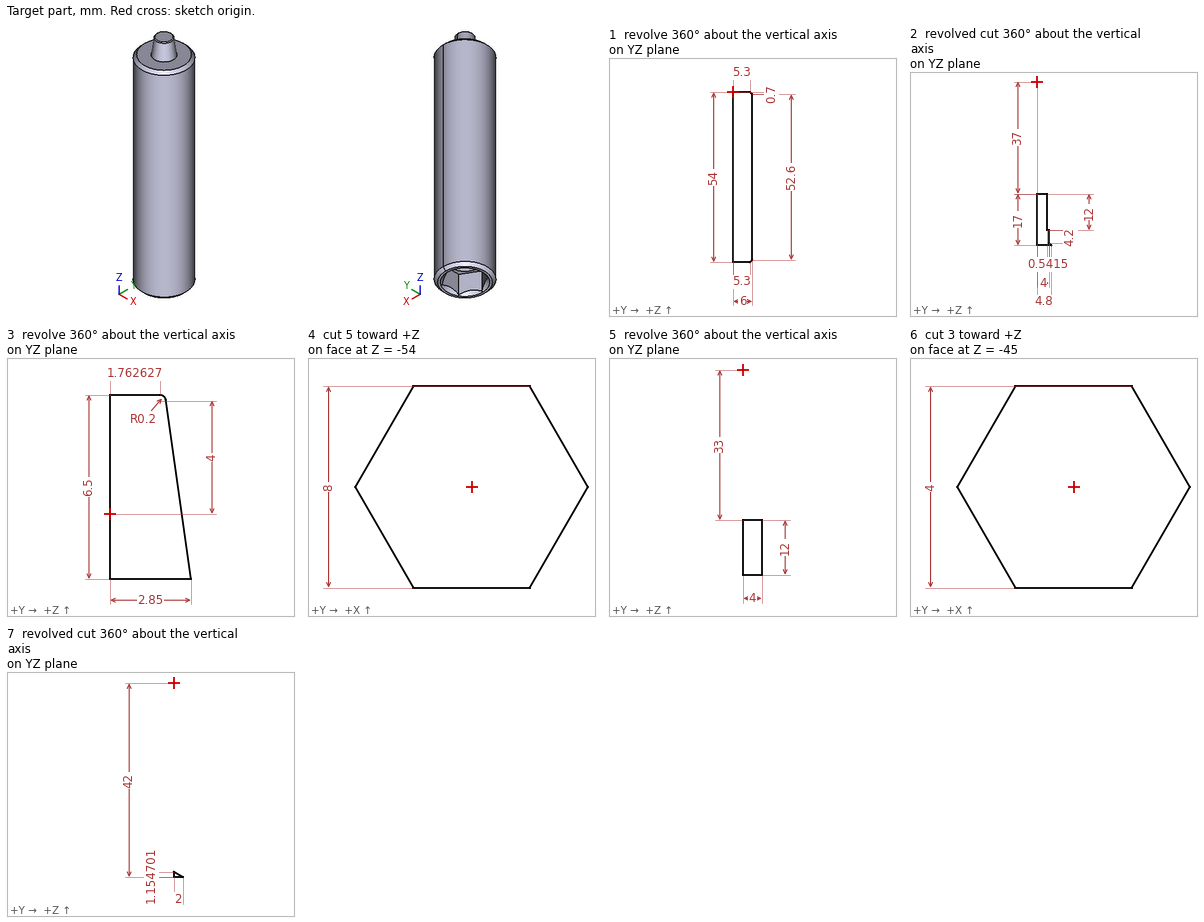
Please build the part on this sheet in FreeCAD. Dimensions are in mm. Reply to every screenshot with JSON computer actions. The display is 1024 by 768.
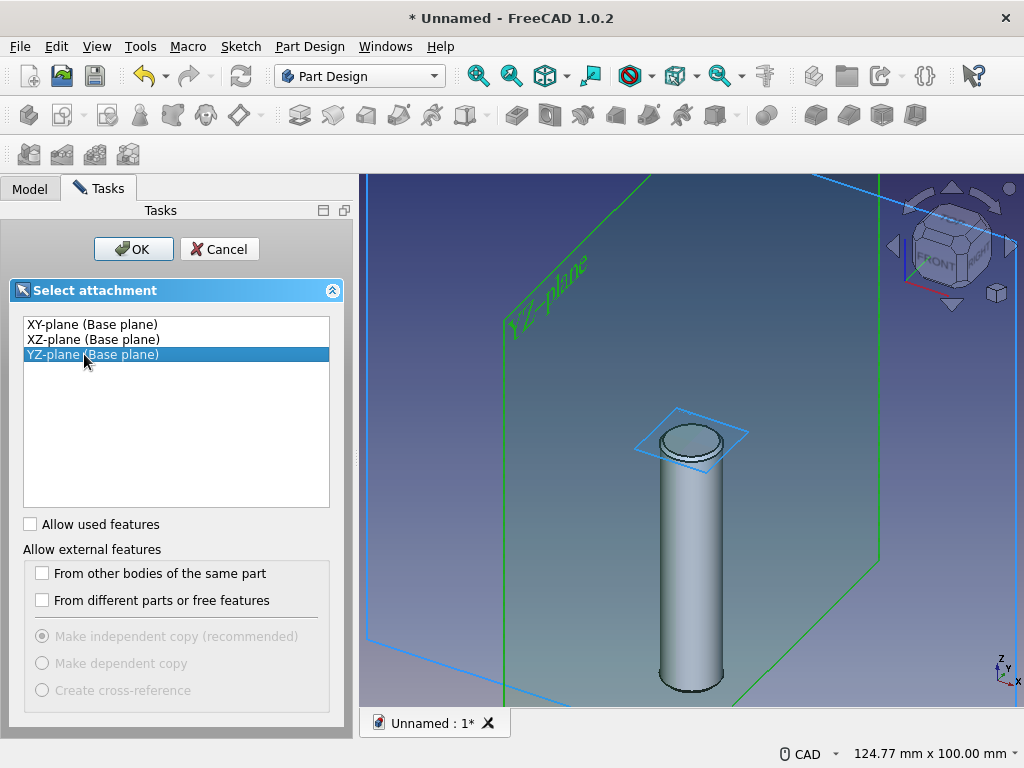
{"action": "left_click", "coordinate": [134, 249]}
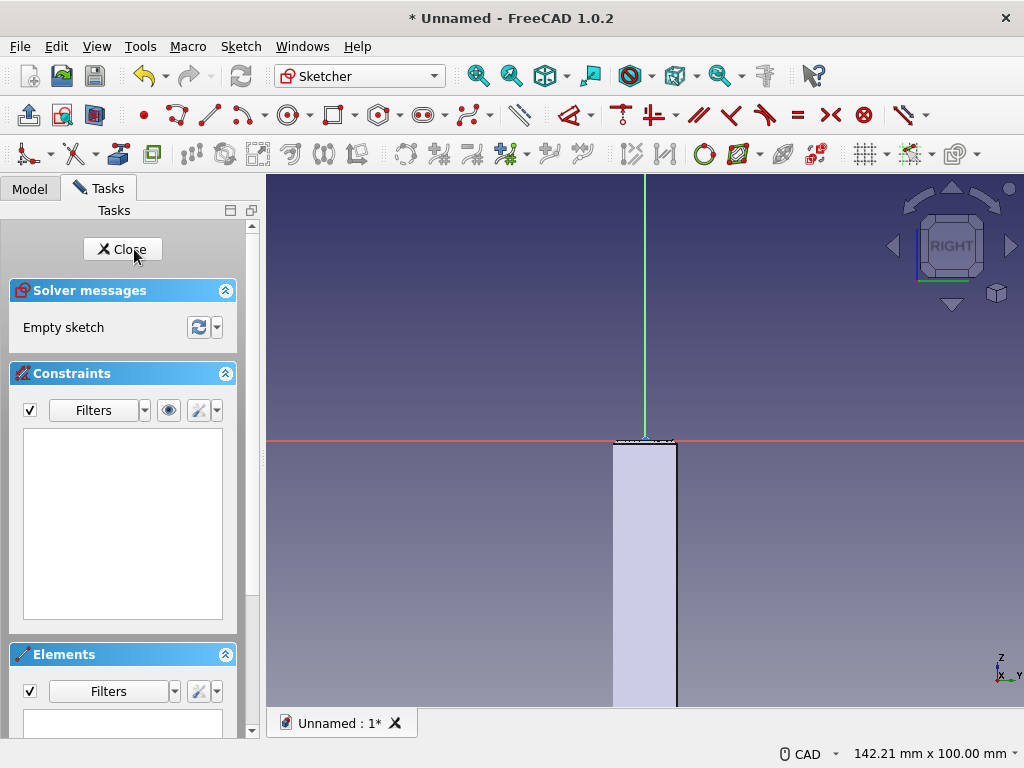
{"action": "left_click", "coordinate": [95, 116]}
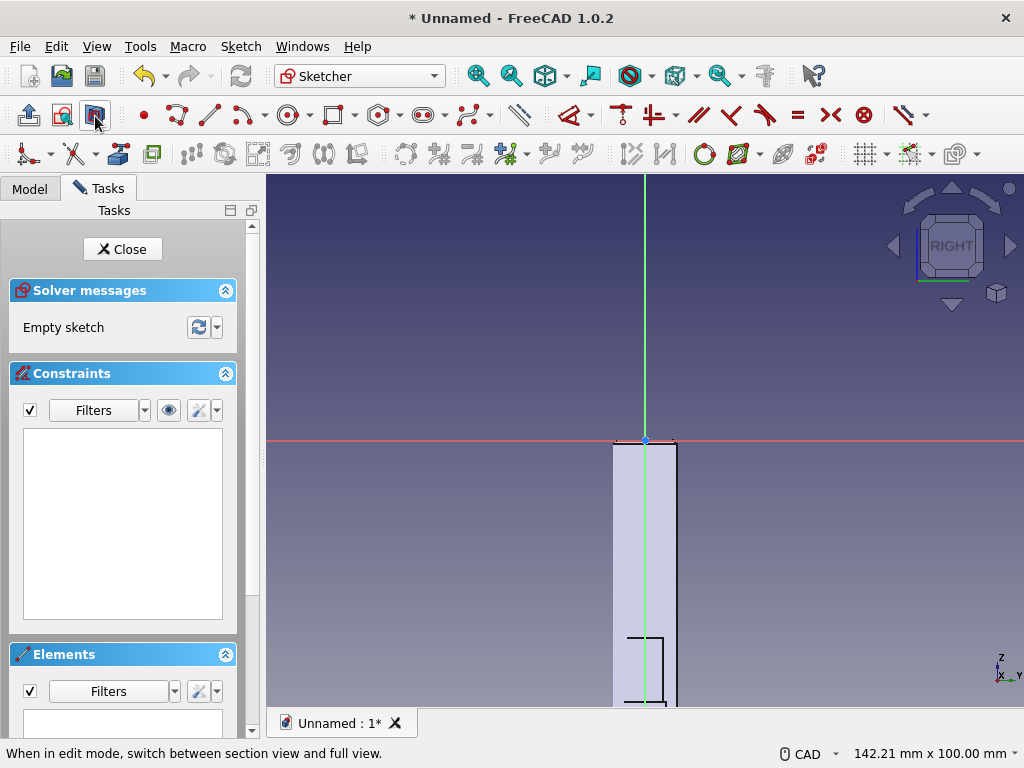
{"action": "scroll", "coordinate": [662, 435], "scroll_direction": "up", "scroll_amount": 11}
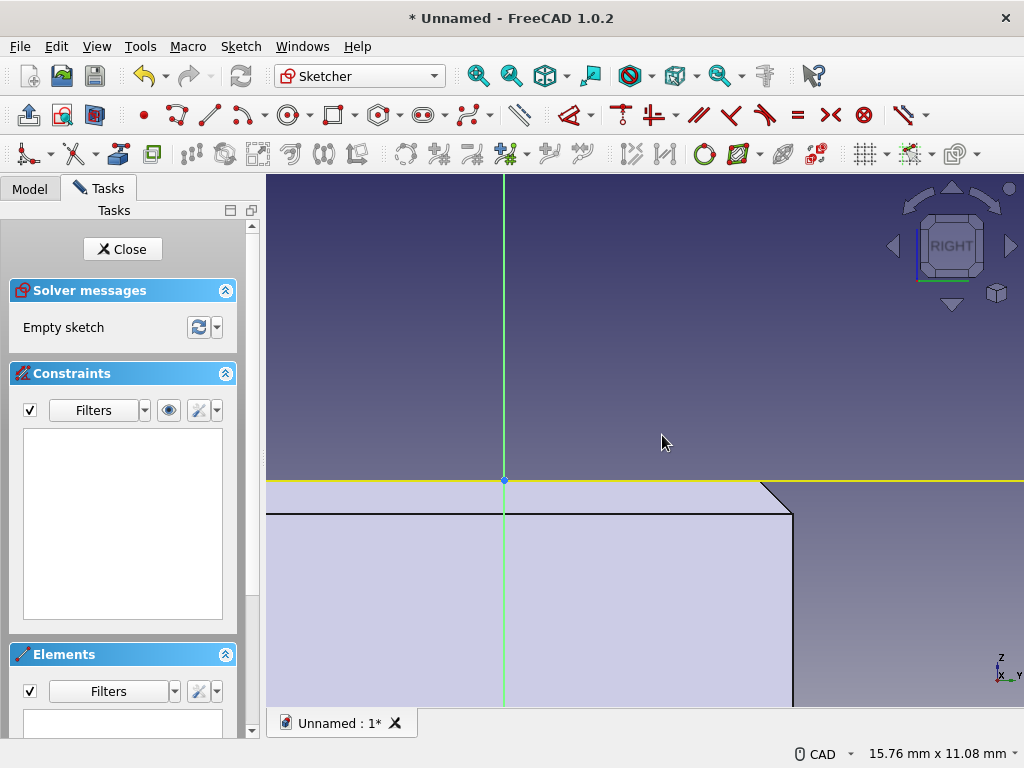
{"action": "left_click", "coordinate": [177, 116]}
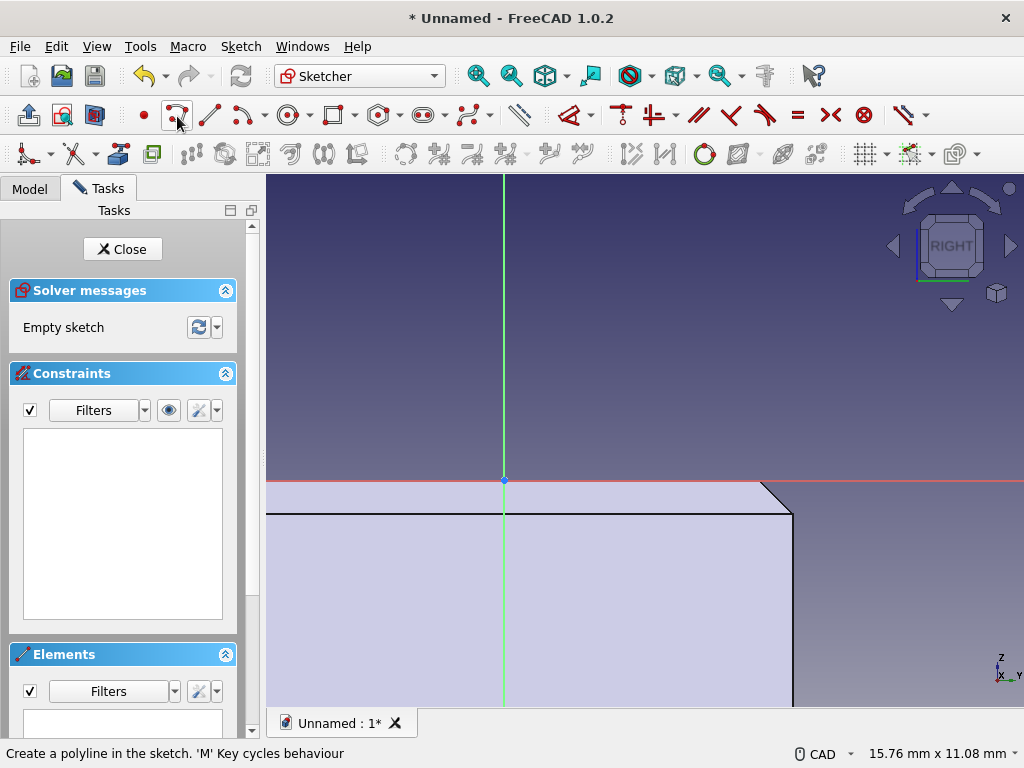
{"action": "left_click", "coordinate": [589, 279]}
{"action": "left_click", "coordinate": [504, 279]}
{"action": "left_click", "coordinate": [513, 591]}
{"action": "left_click", "coordinate": [641, 591]}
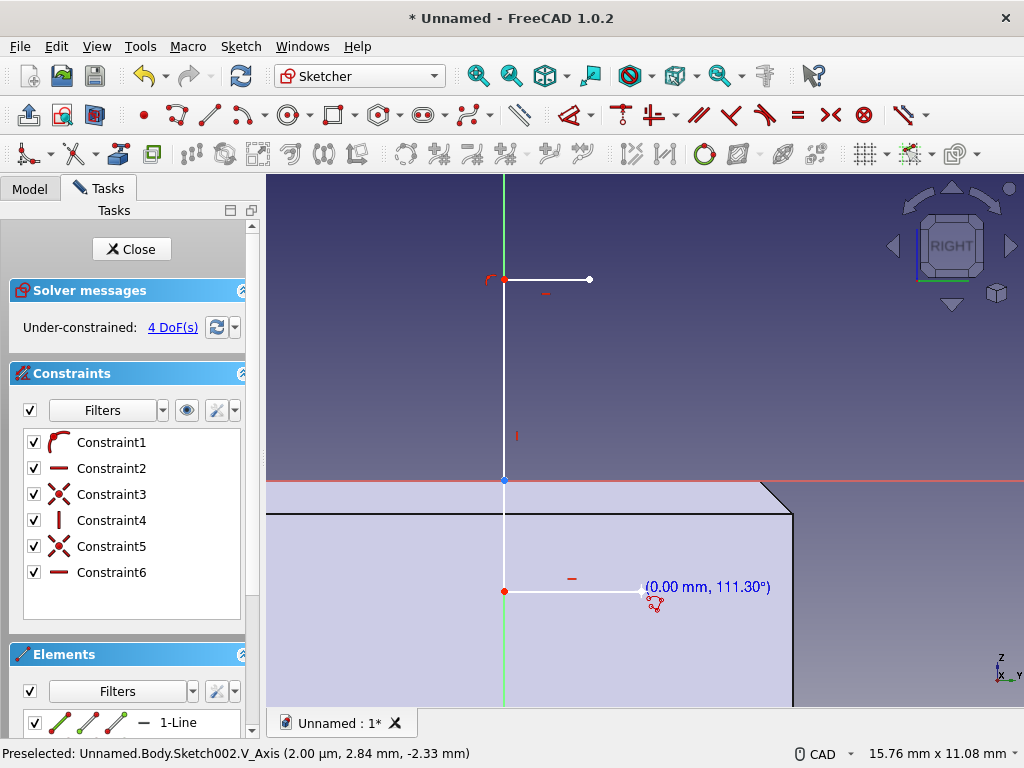
{"action": "scroll", "coordinate": [599, 287], "scroll_direction": "up", "scroll_amount": 2}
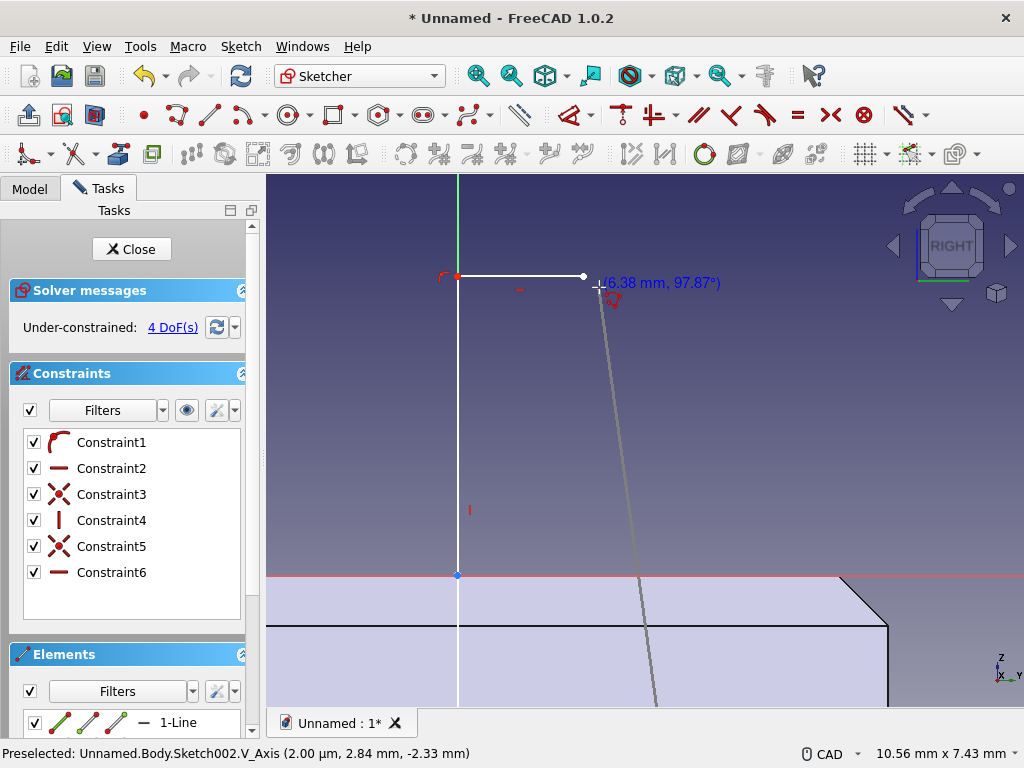
{"action": "left_click", "coordinate": [598, 287]}
{"action": "right_click", "coordinate": [598, 287]}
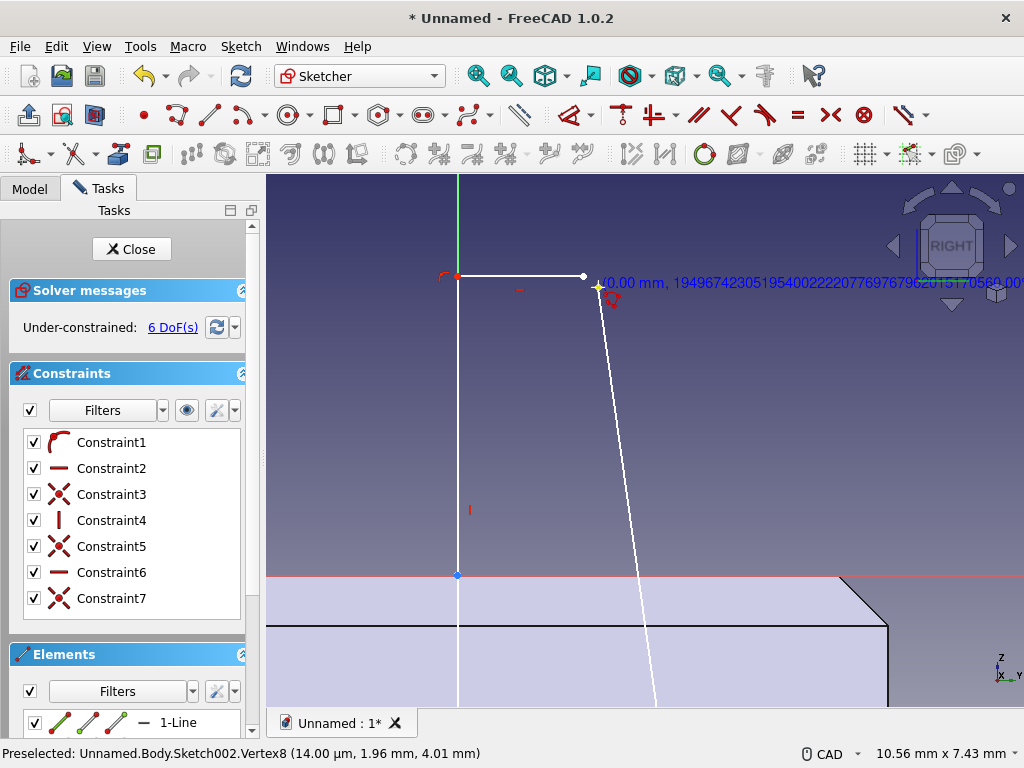
{"action": "left_click", "coordinate": [264, 116]}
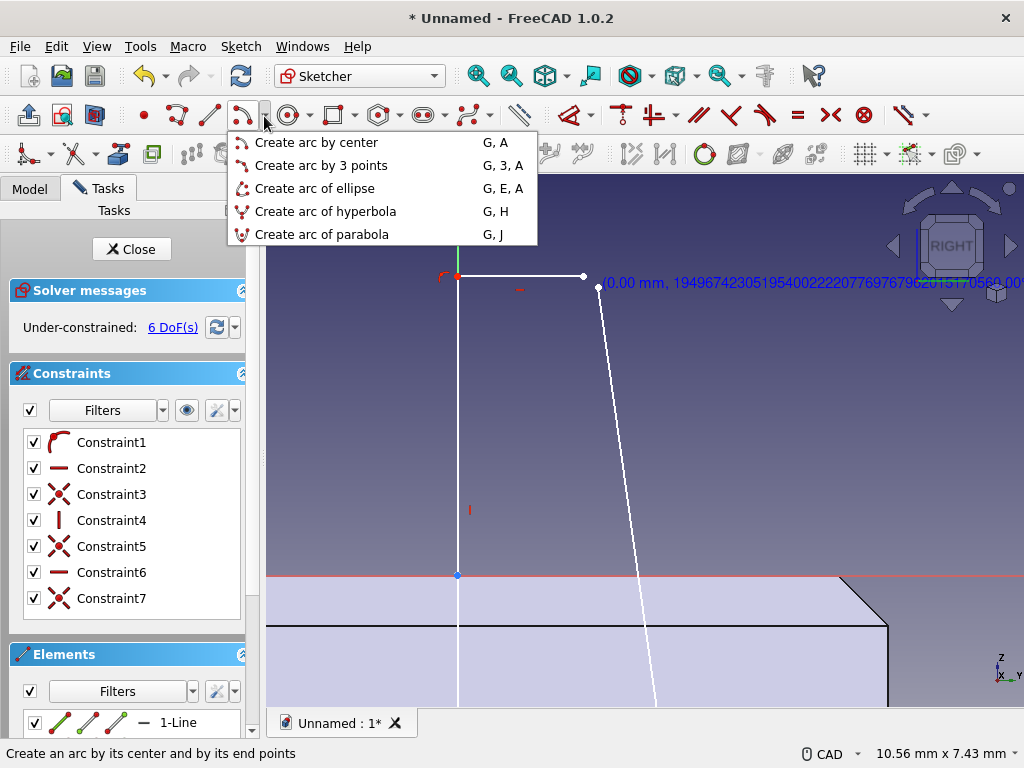
{"action": "left_click", "coordinate": [382, 166]}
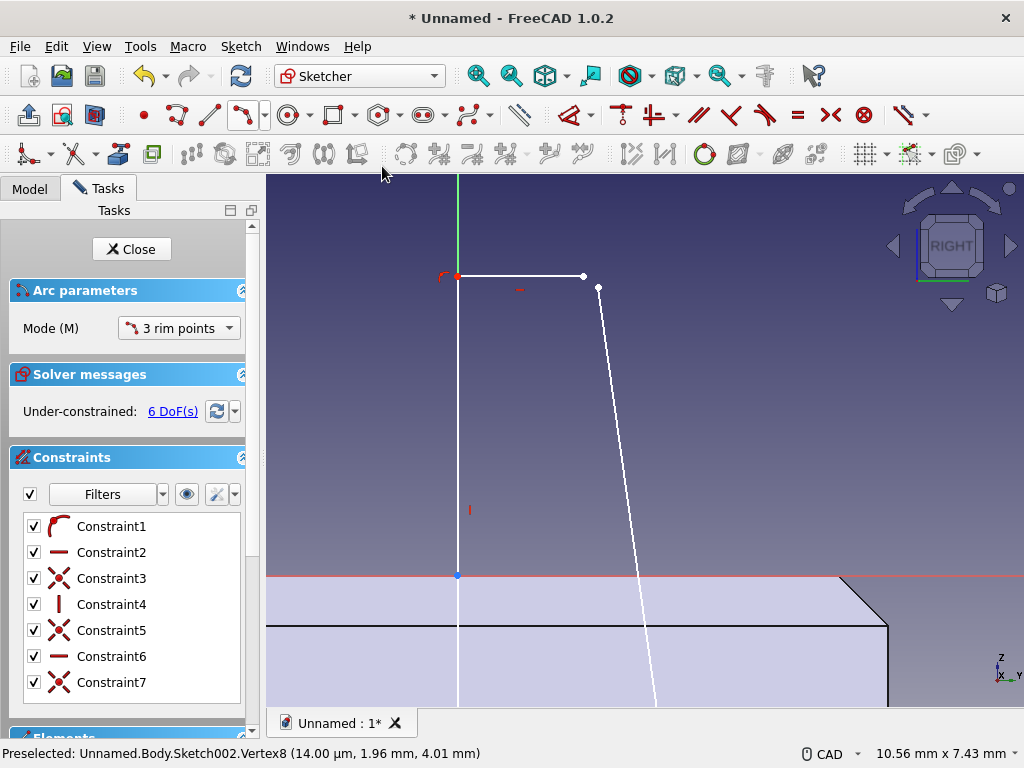
{"action": "left_click", "coordinate": [598, 288]}
{"action": "left_click", "coordinate": [584, 276]}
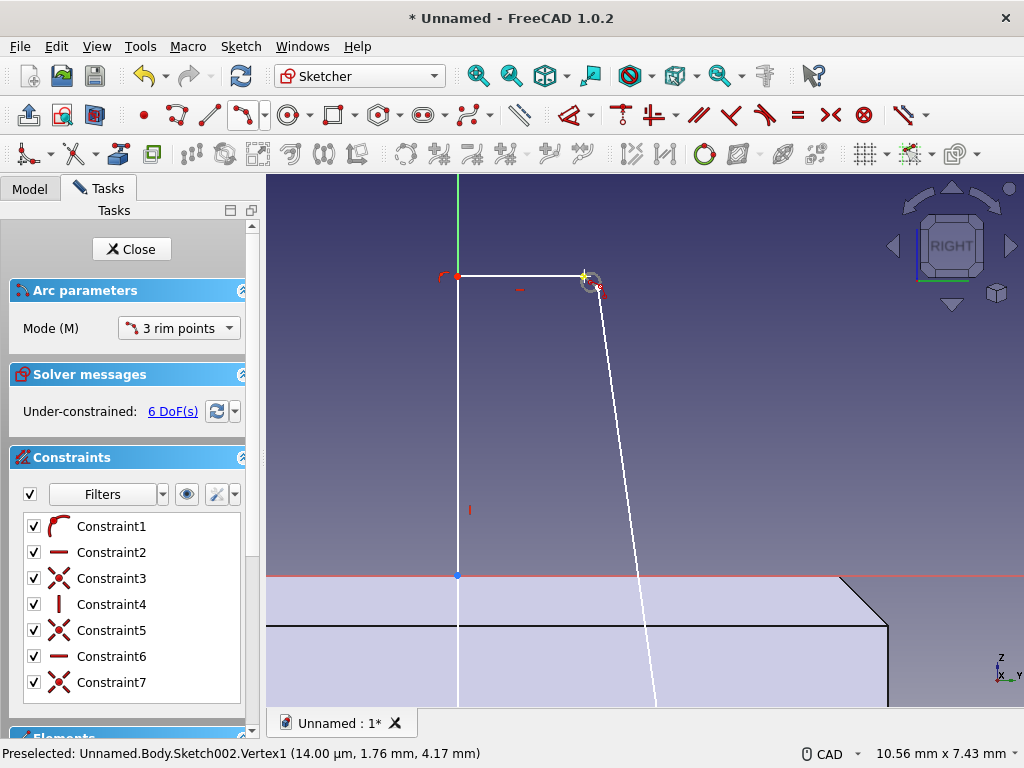
{"action": "scroll", "coordinate": [594, 278], "scroll_direction": "up", "scroll_amount": 8}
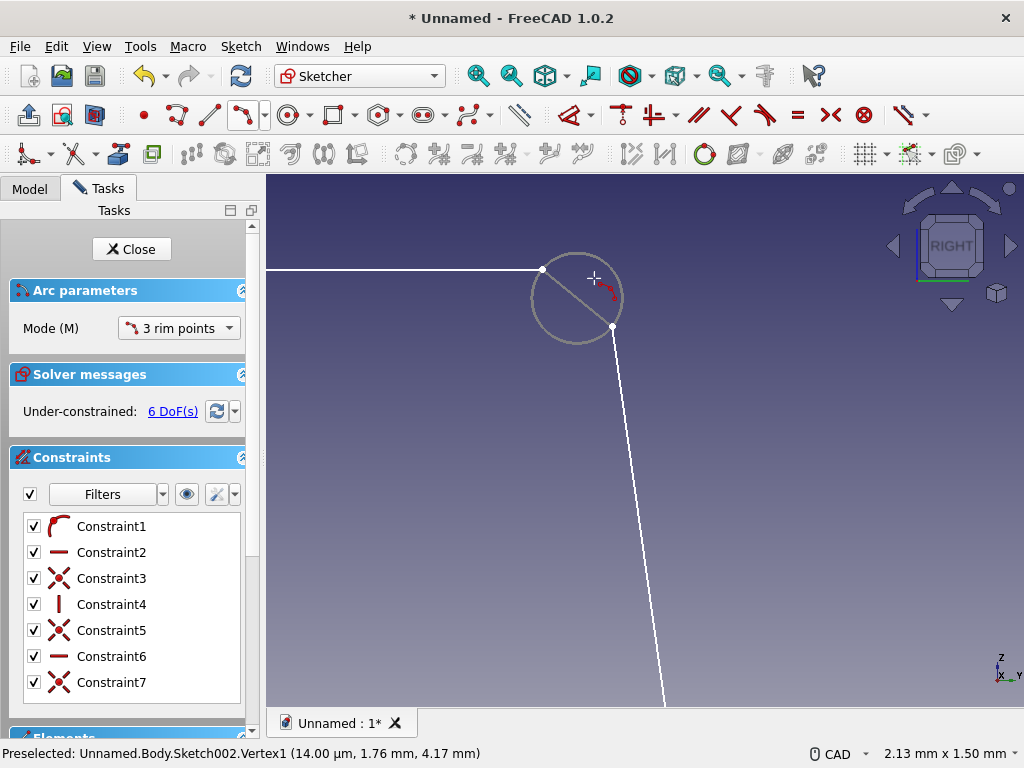
{"action": "left_click", "coordinate": [590, 277]}
{"action": "key", "text": "Escape"}